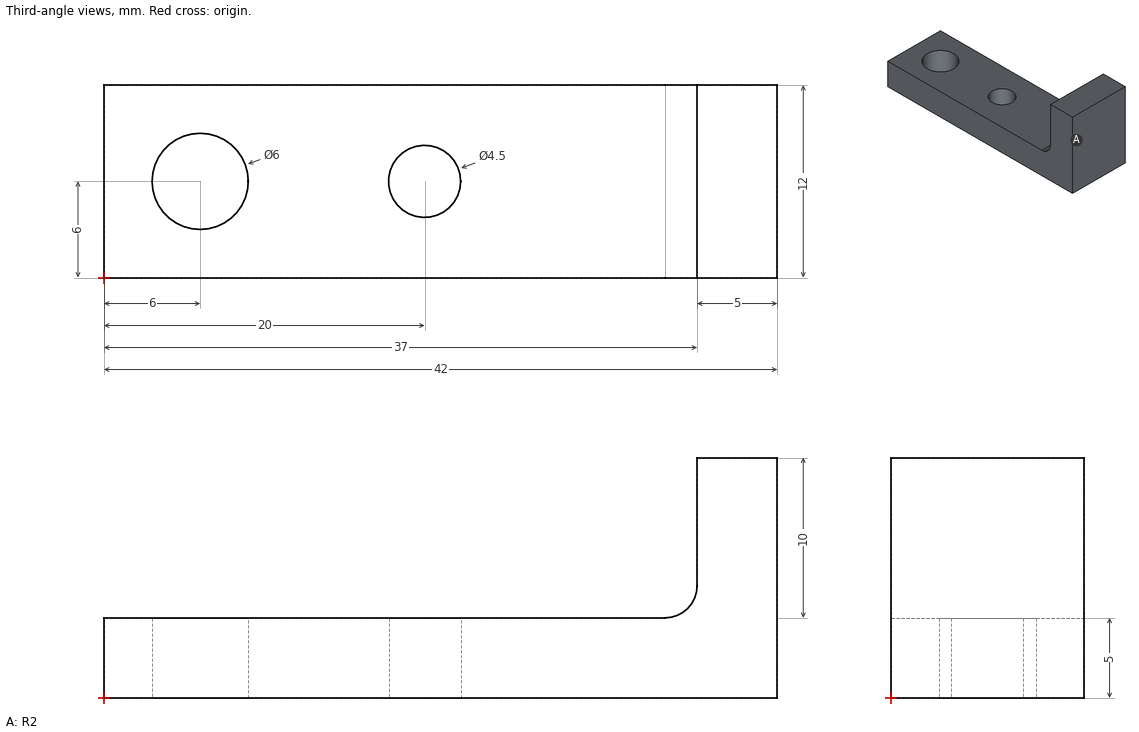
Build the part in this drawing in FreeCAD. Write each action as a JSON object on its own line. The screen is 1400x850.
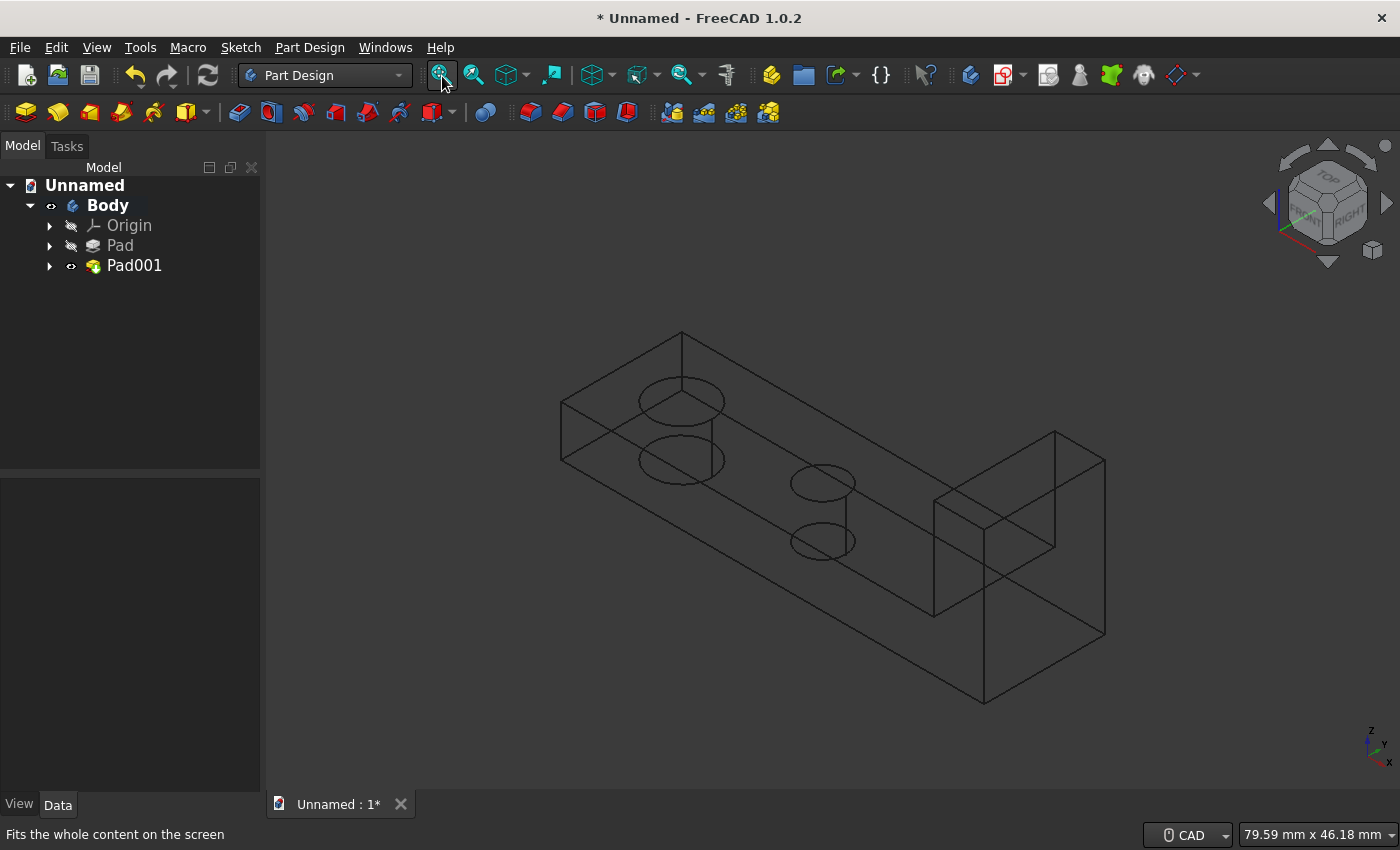
{"action": "left_click", "coordinate": [994, 581]}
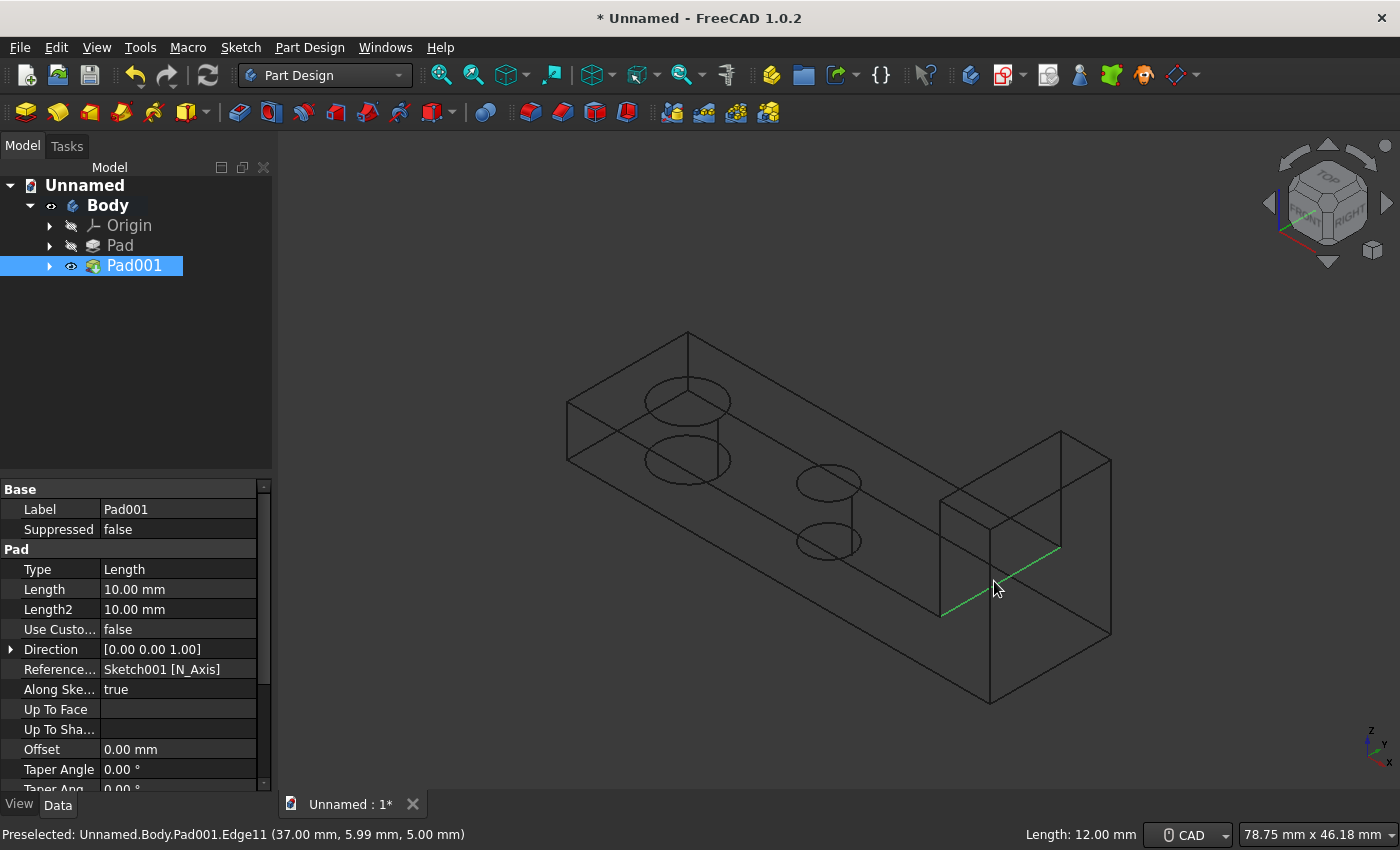
{"action": "key", "text": "v 1"}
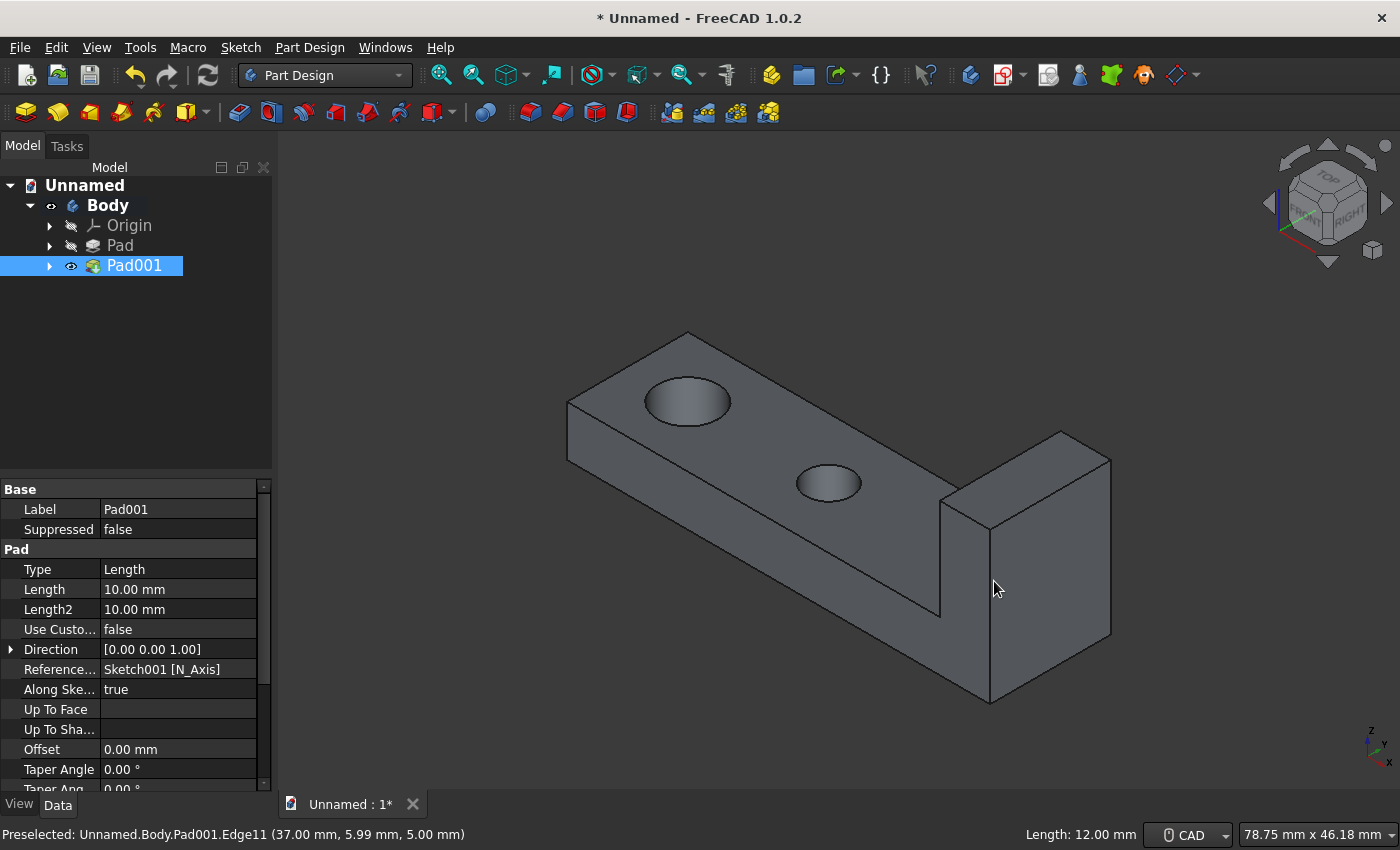
{"action": "left_click", "coordinate": [532, 112]}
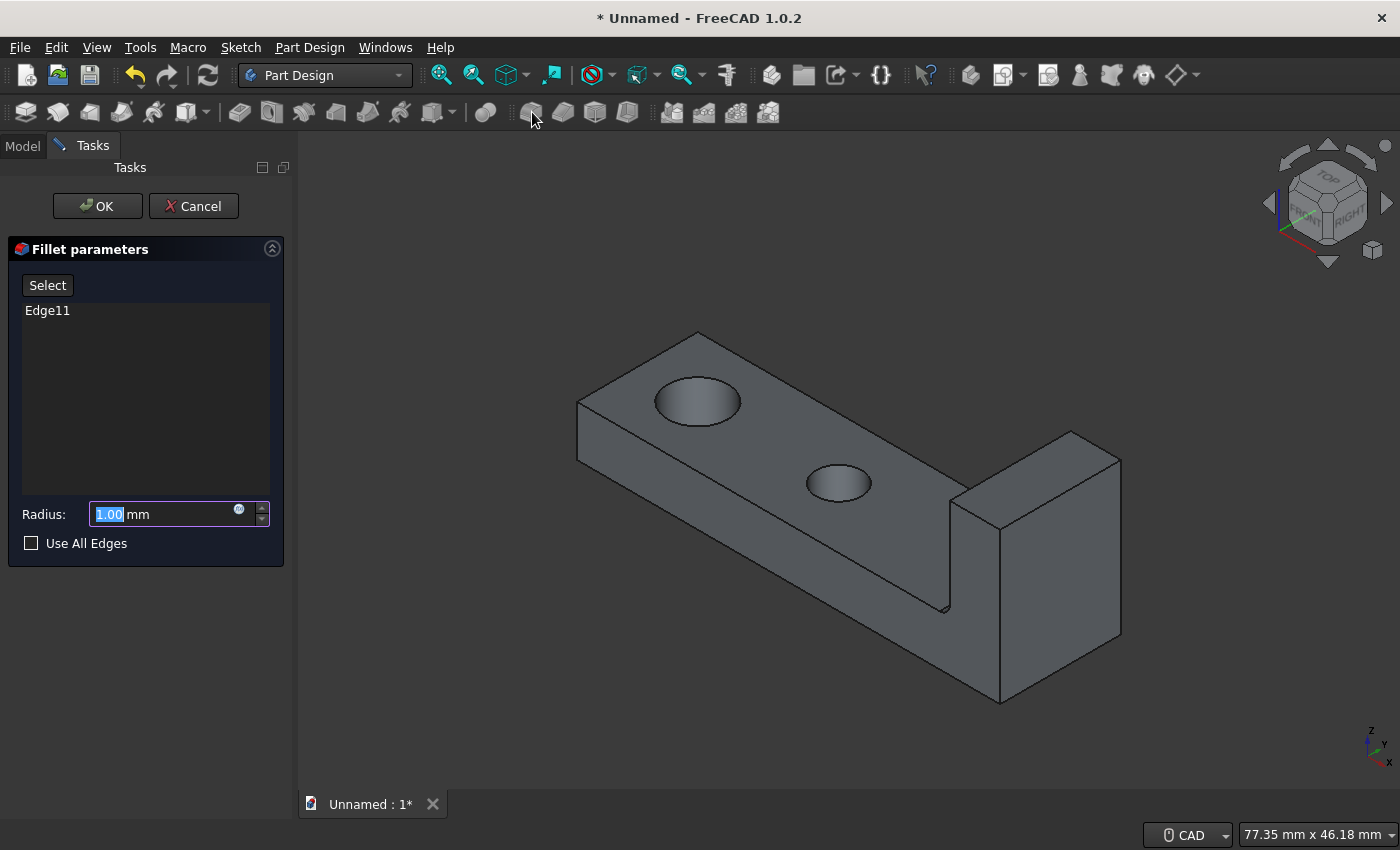
{"action": "type", "text": "2"}
{"action": "key", "text": "Tab"}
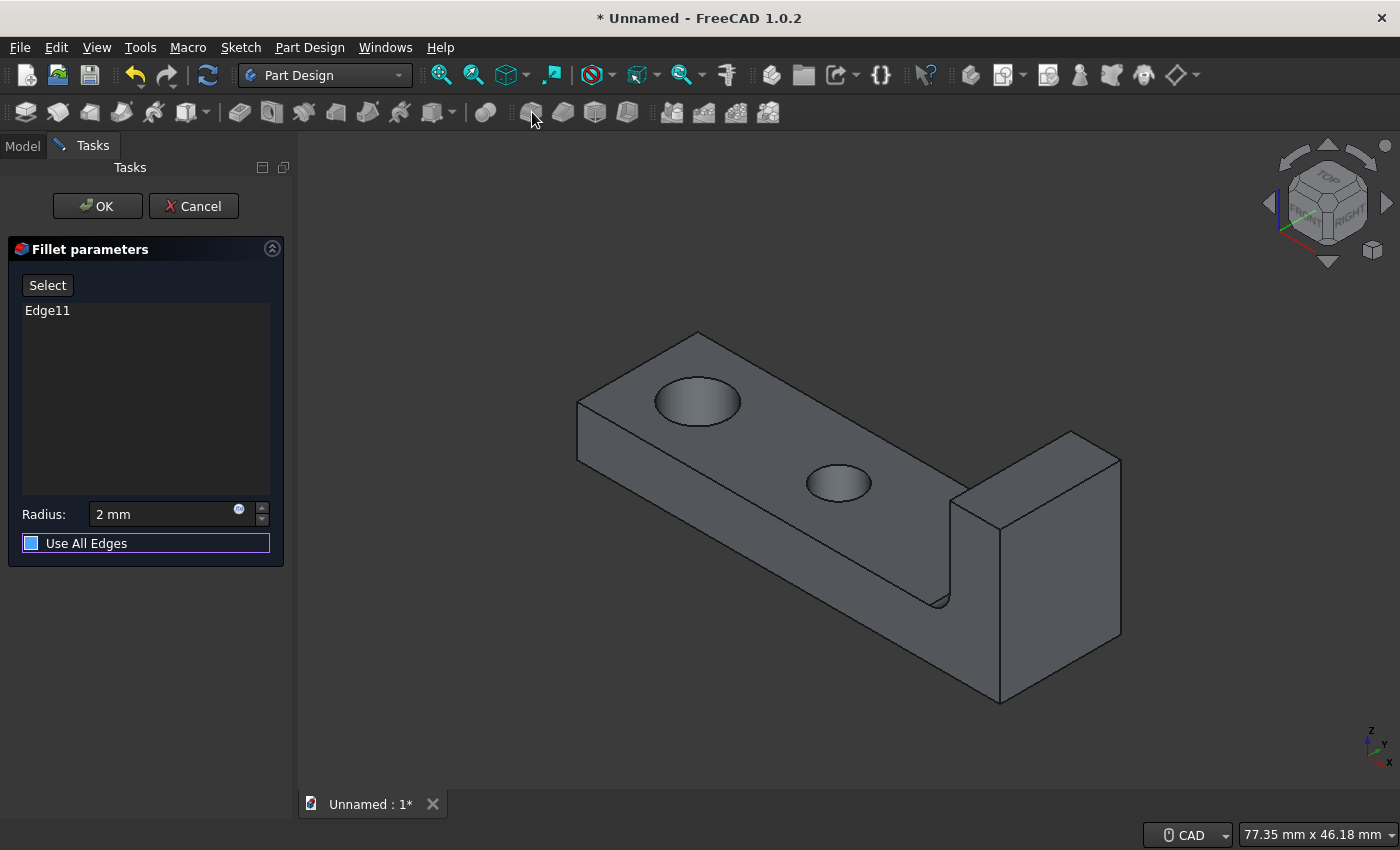
{"action": "left_click", "coordinate": [98, 206]}